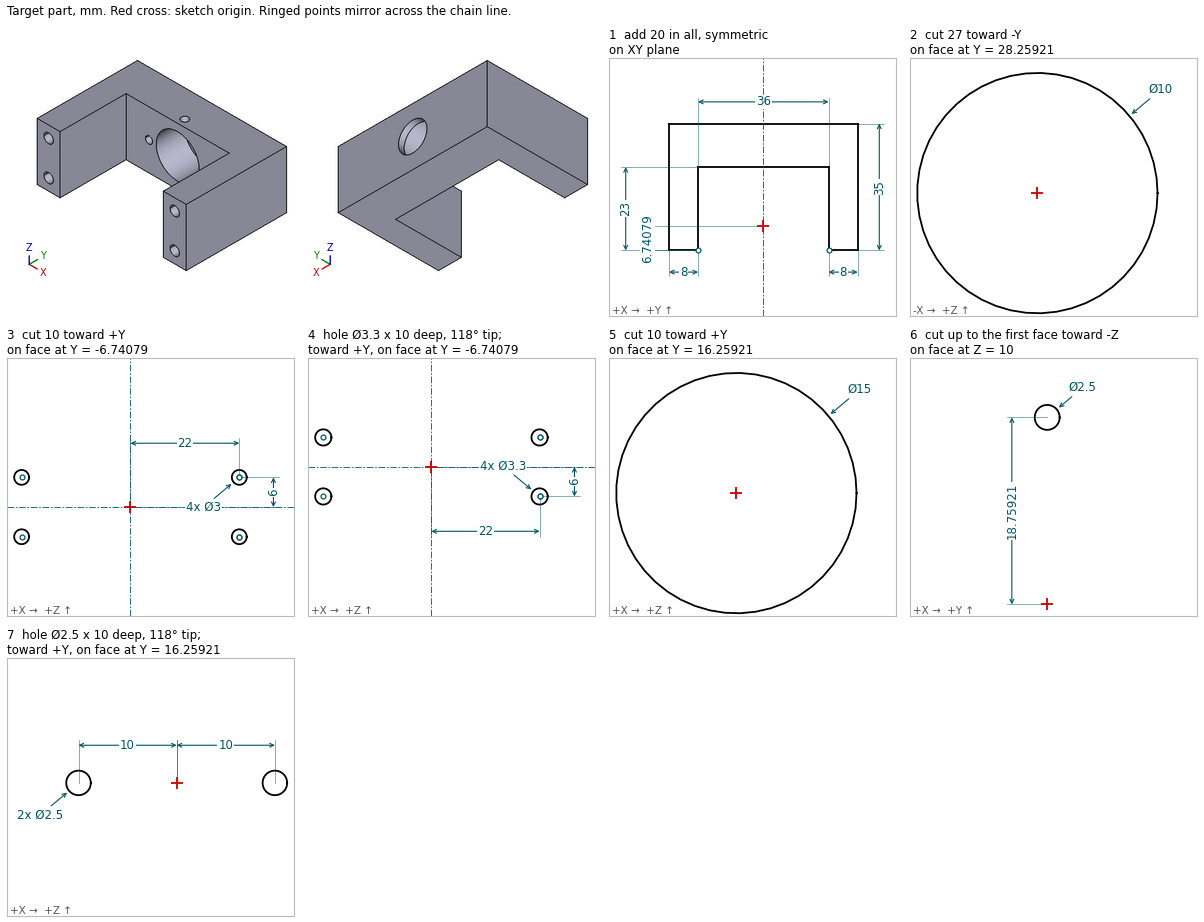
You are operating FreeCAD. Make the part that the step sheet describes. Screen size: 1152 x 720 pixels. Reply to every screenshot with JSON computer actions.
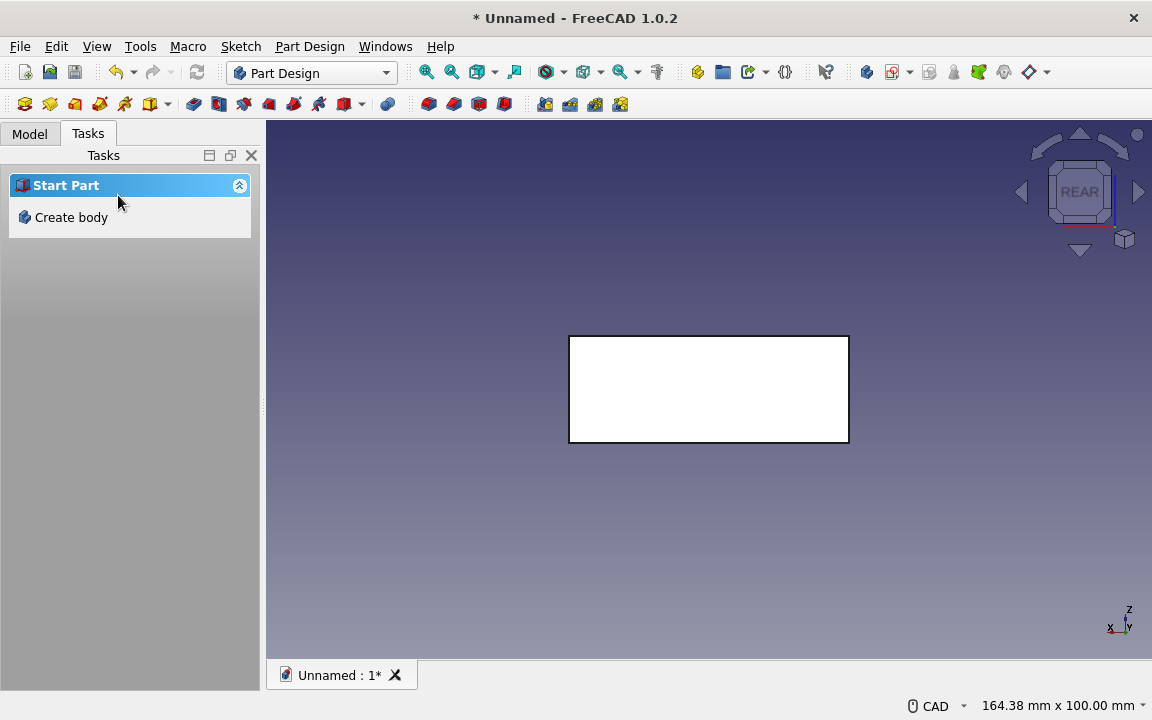
{"action": "key", "text": "v f"}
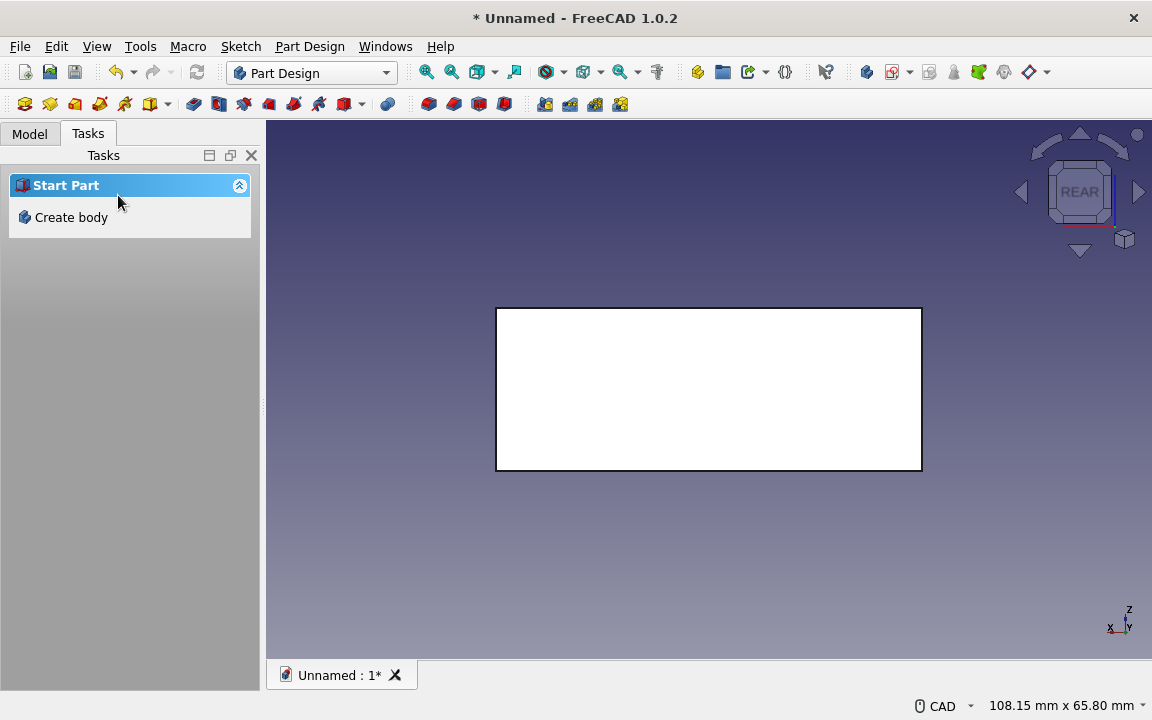
{"action": "left_click", "coordinate": [587, 389]}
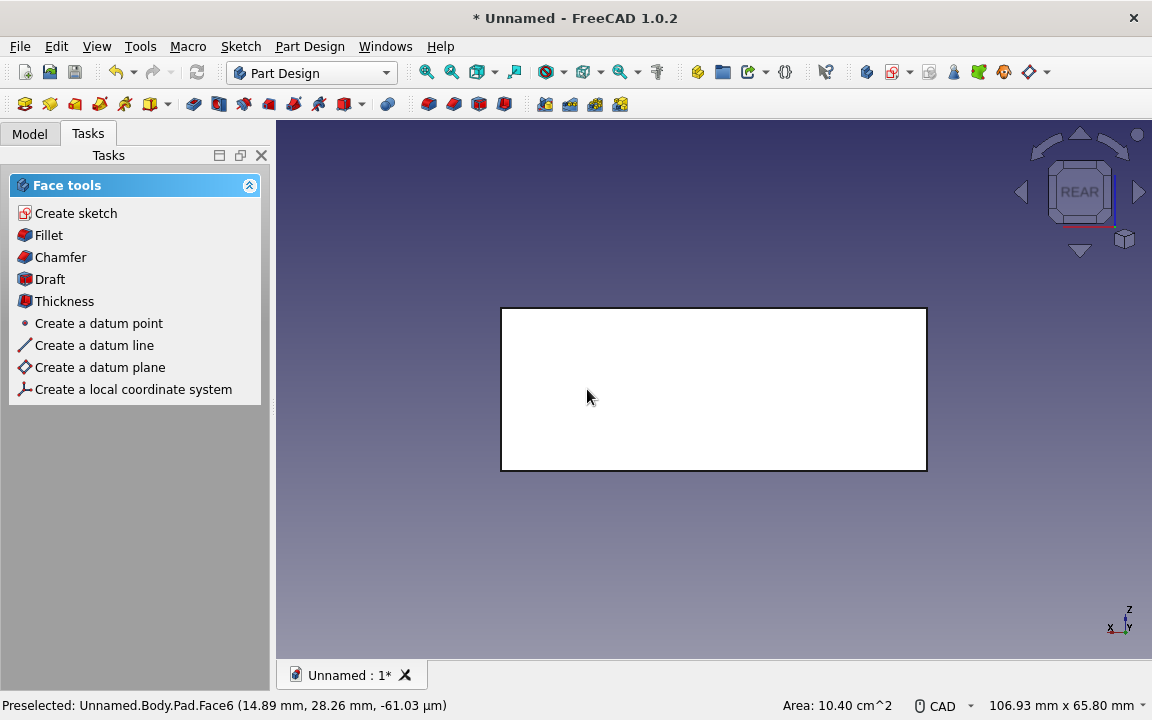
{"action": "left_click", "coordinate": [892, 72]}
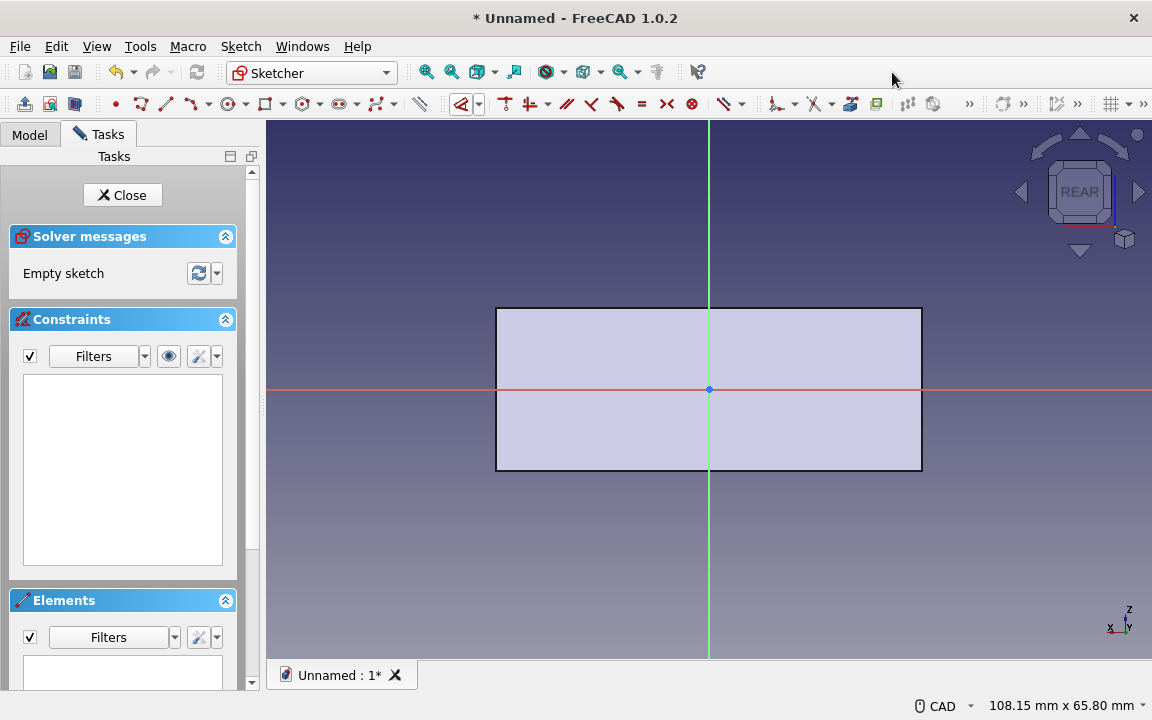
{"action": "scroll", "coordinate": [731, 390], "scroll_direction": "up", "scroll_amount": 7}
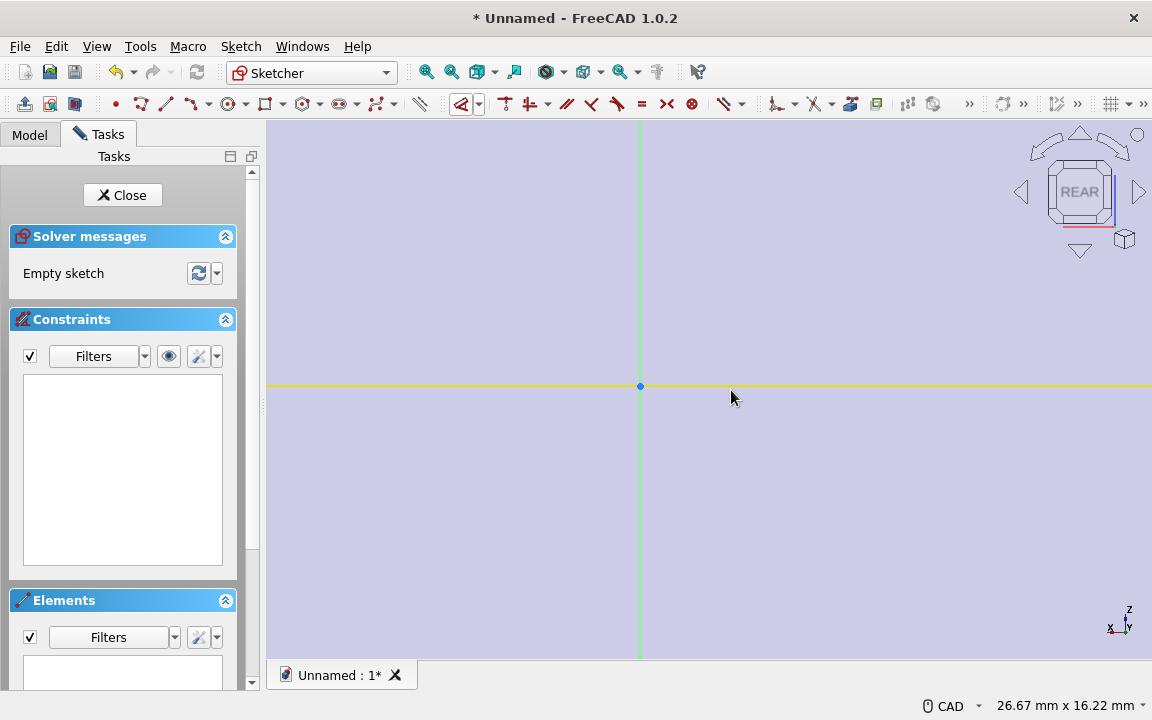
{"action": "key", "text": "g c"}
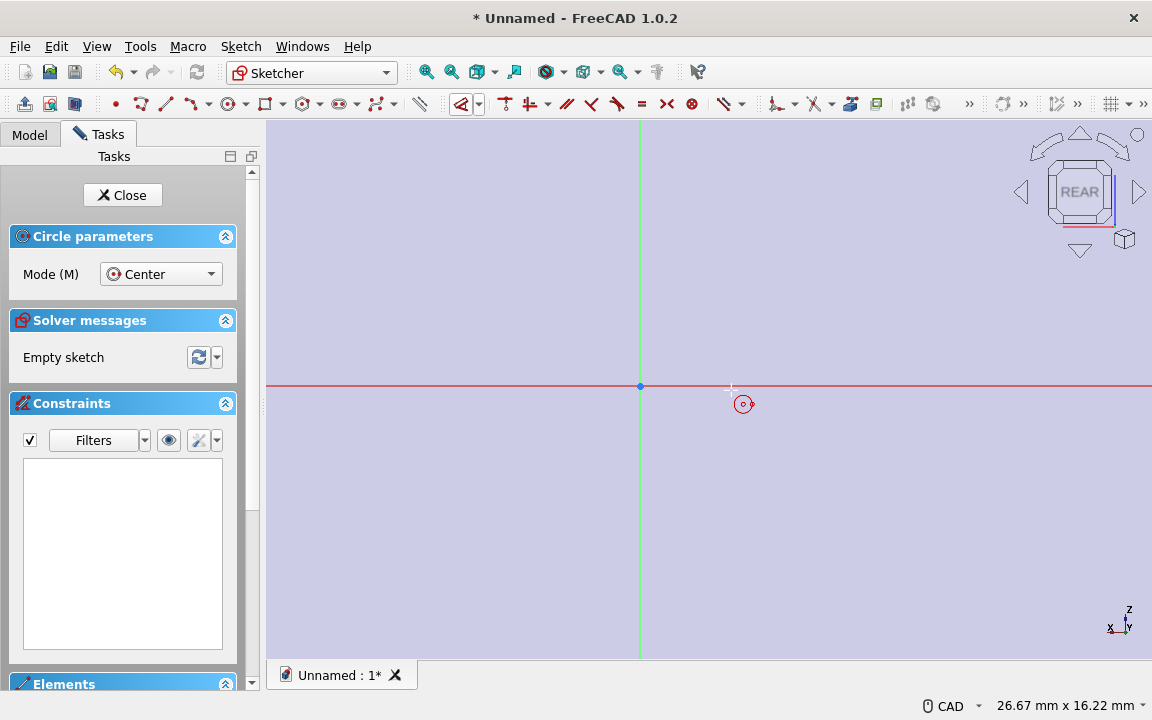
{"action": "left_click", "coordinate": [640, 386]}
{"action": "left_click", "coordinate": [758, 269]}
{"action": "key", "text": "Escape"}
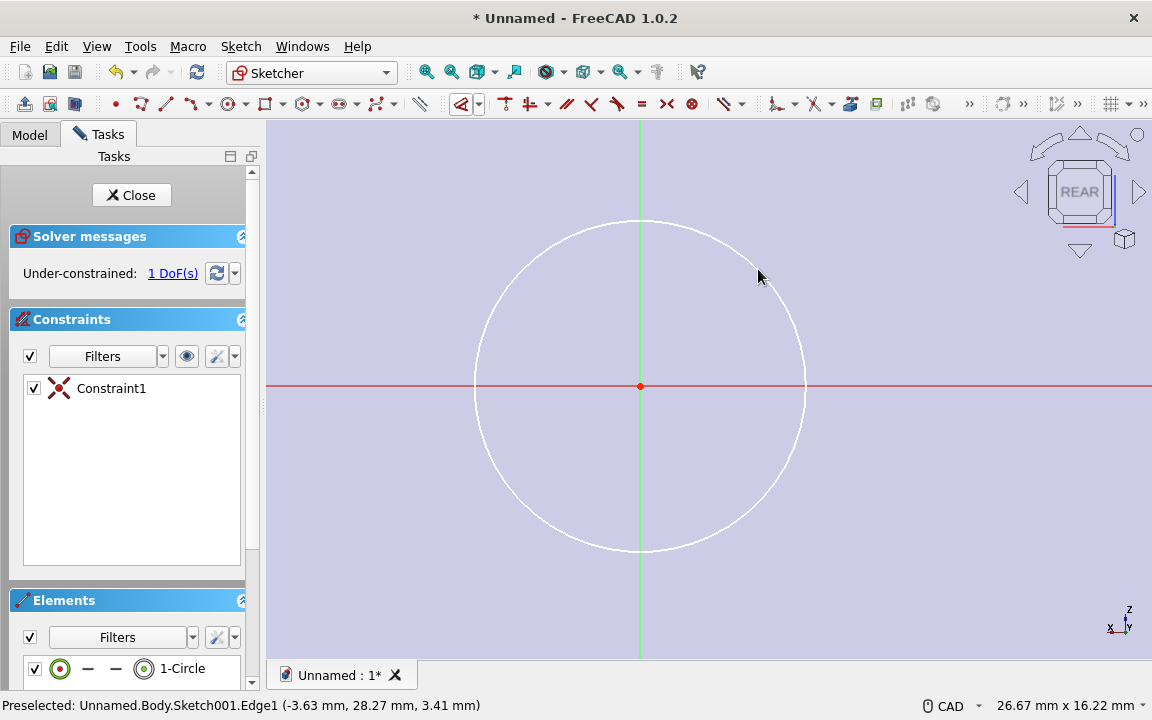
{"action": "left_click", "coordinate": [757, 269]}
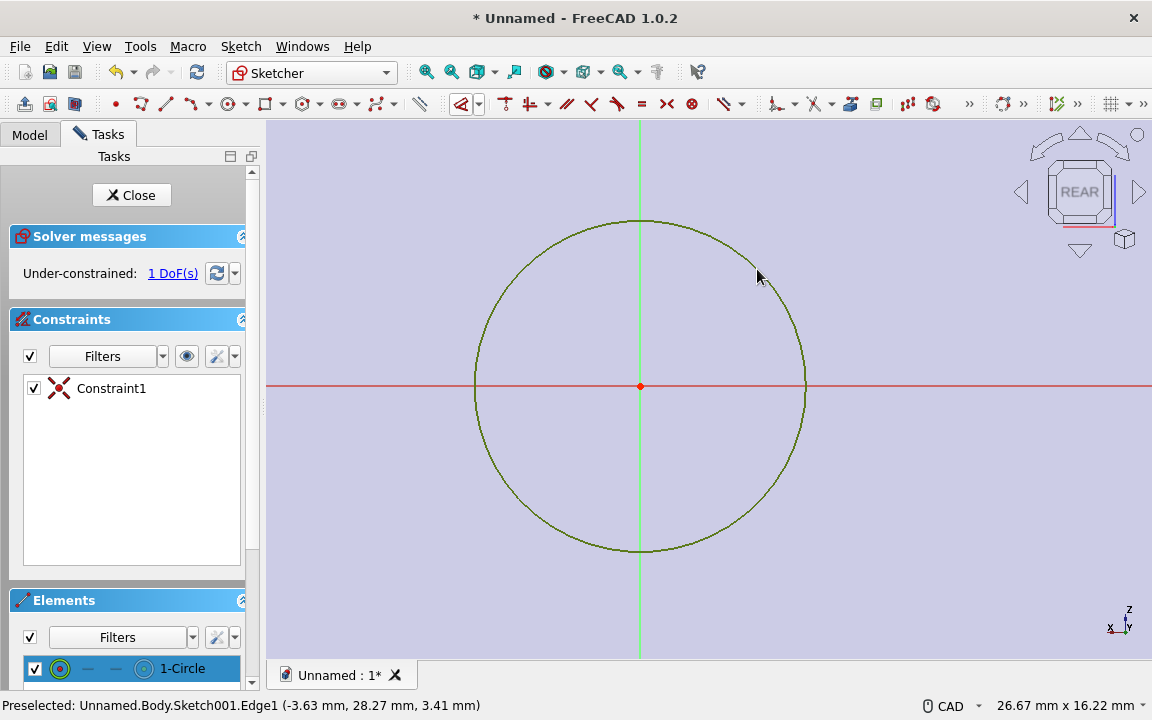
{"action": "key", "text": "k o"}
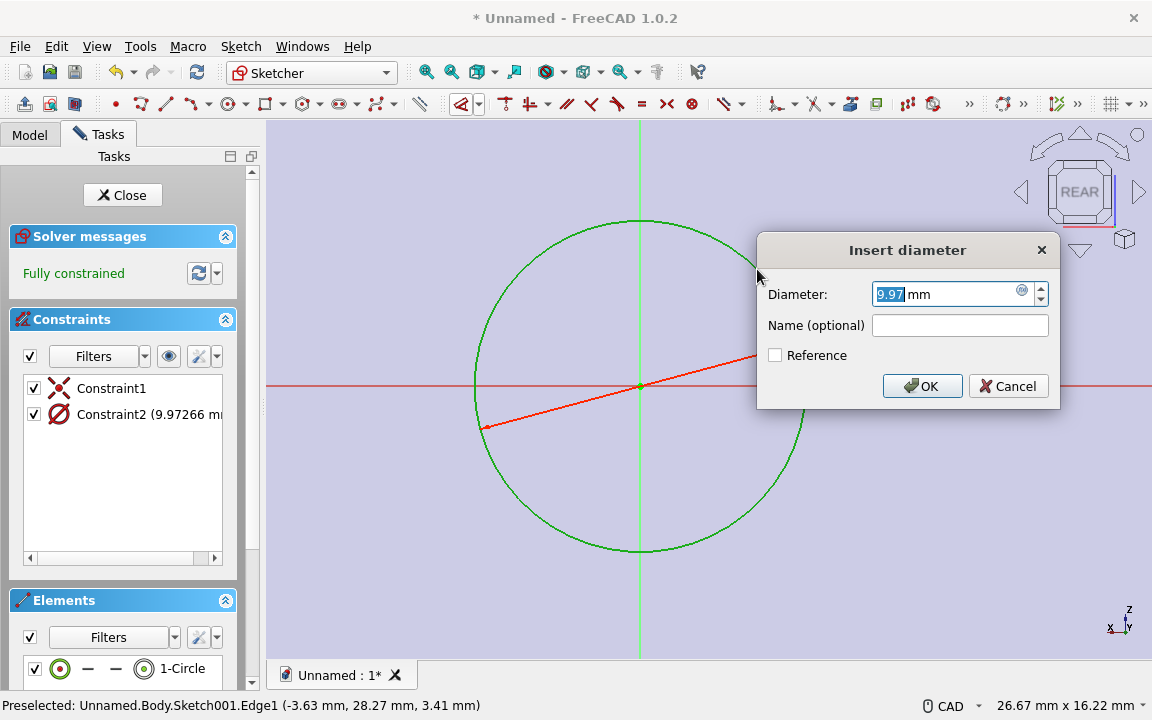
{"action": "type", "text": "10"}
{"action": "key", "text": "Return"}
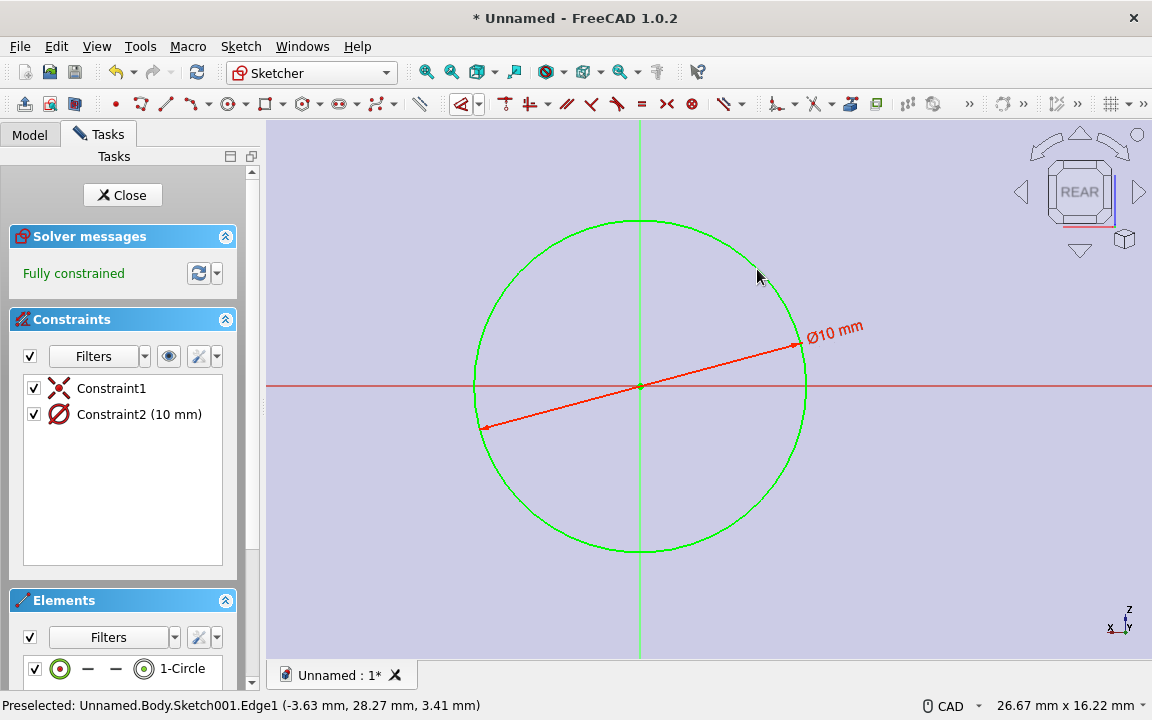
{"action": "left_click", "coordinate": [123, 195]}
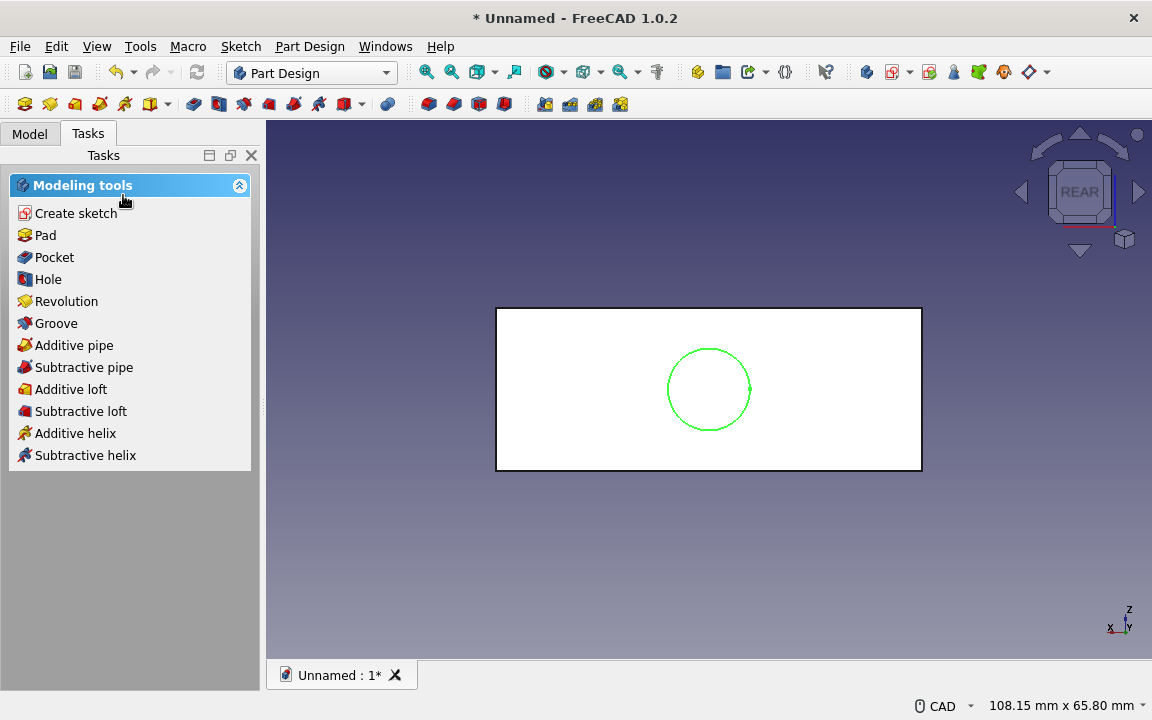
{"action": "left_click", "coordinate": [194, 104]}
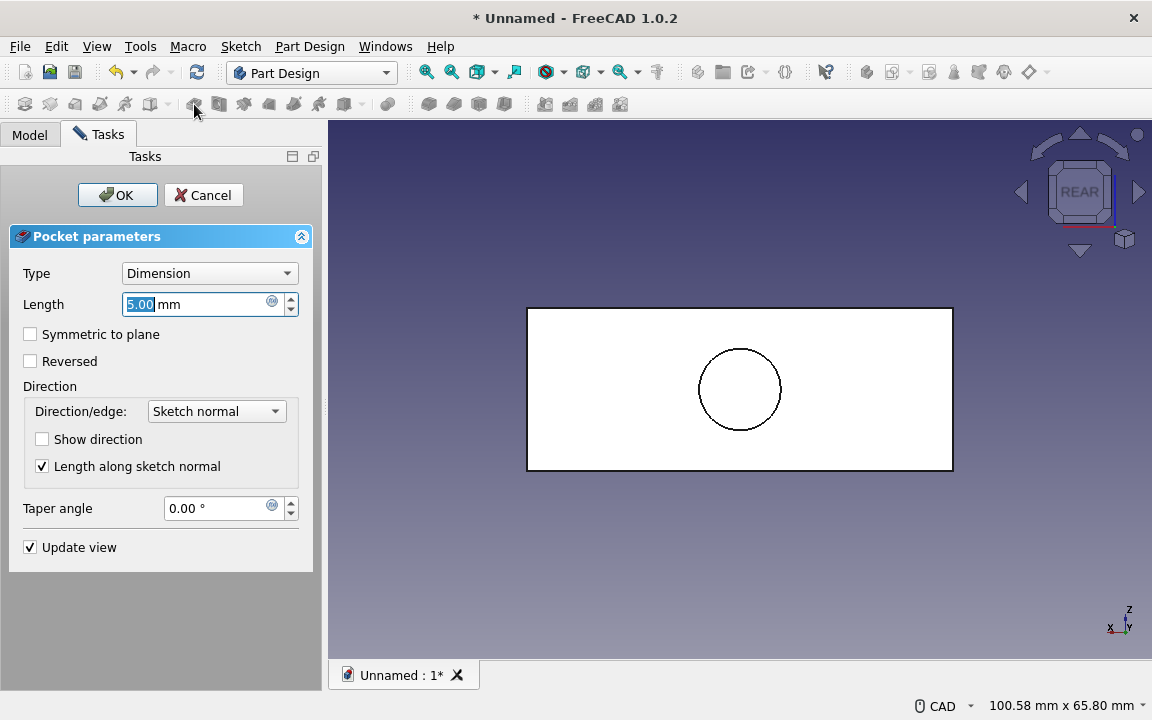
{"action": "type", "text": "27"}
{"action": "key", "text": "Tab"}